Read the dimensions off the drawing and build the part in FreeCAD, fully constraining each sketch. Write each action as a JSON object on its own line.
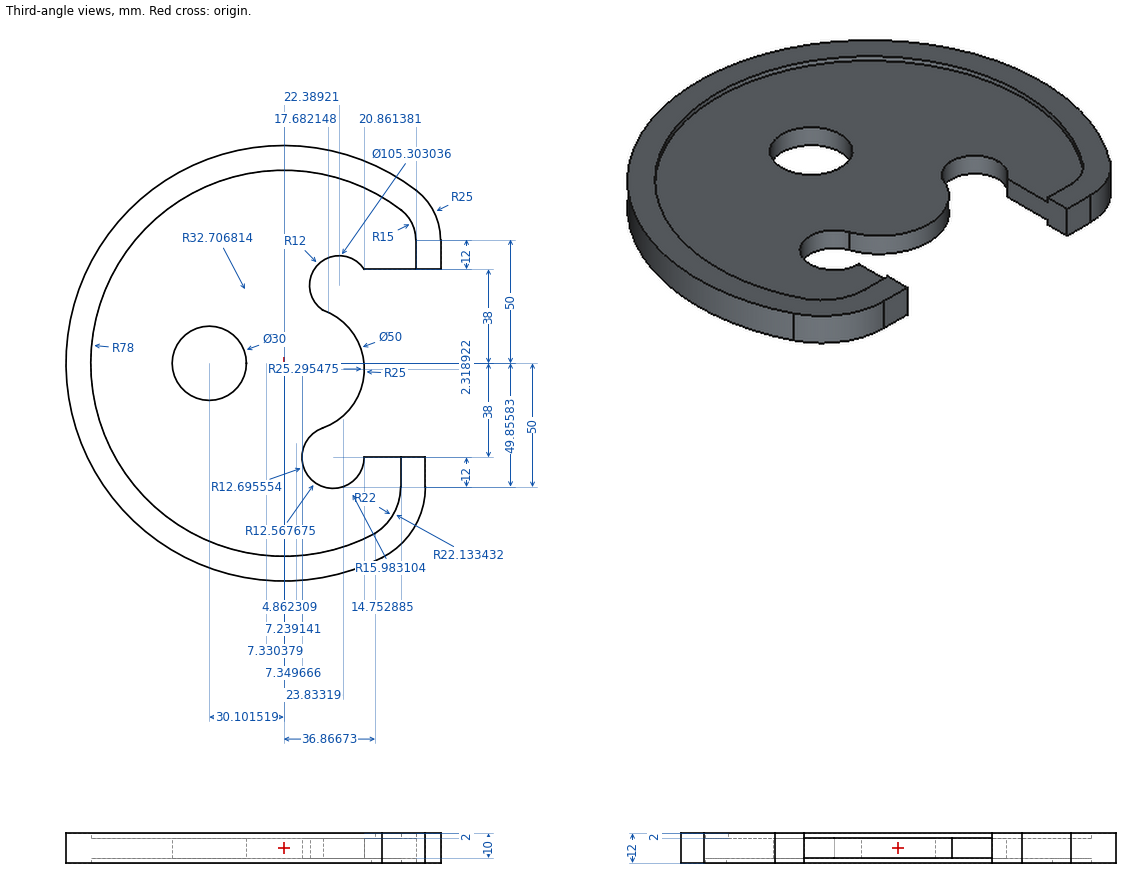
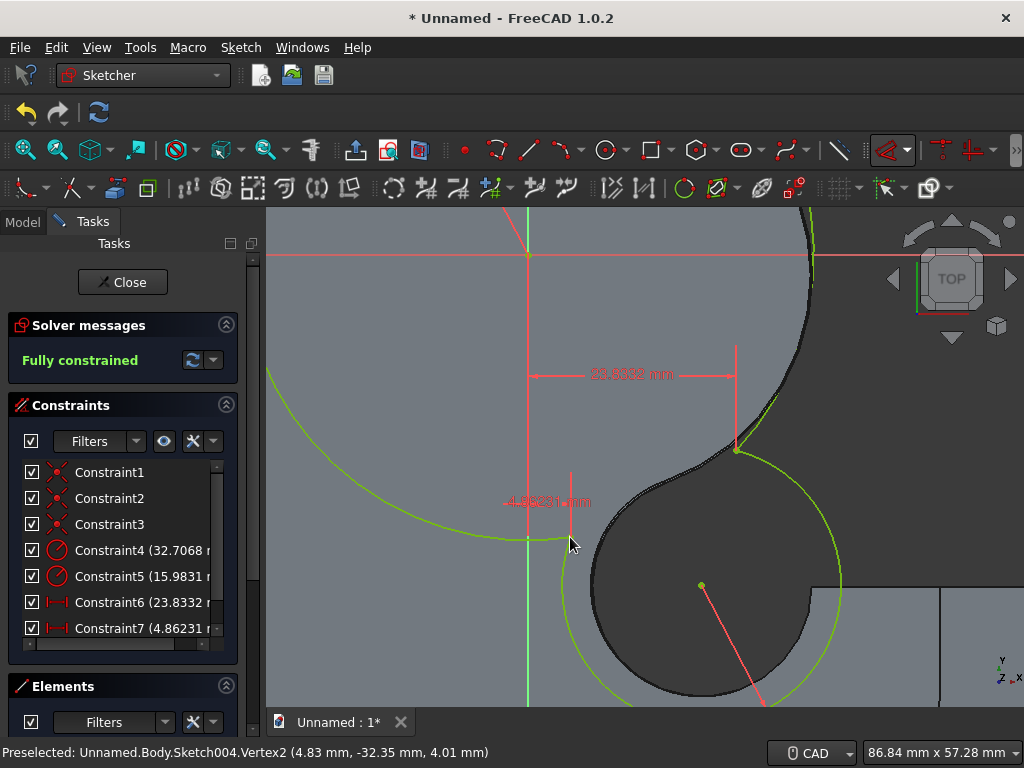
{"action": "left_click", "coordinate": [123, 282]}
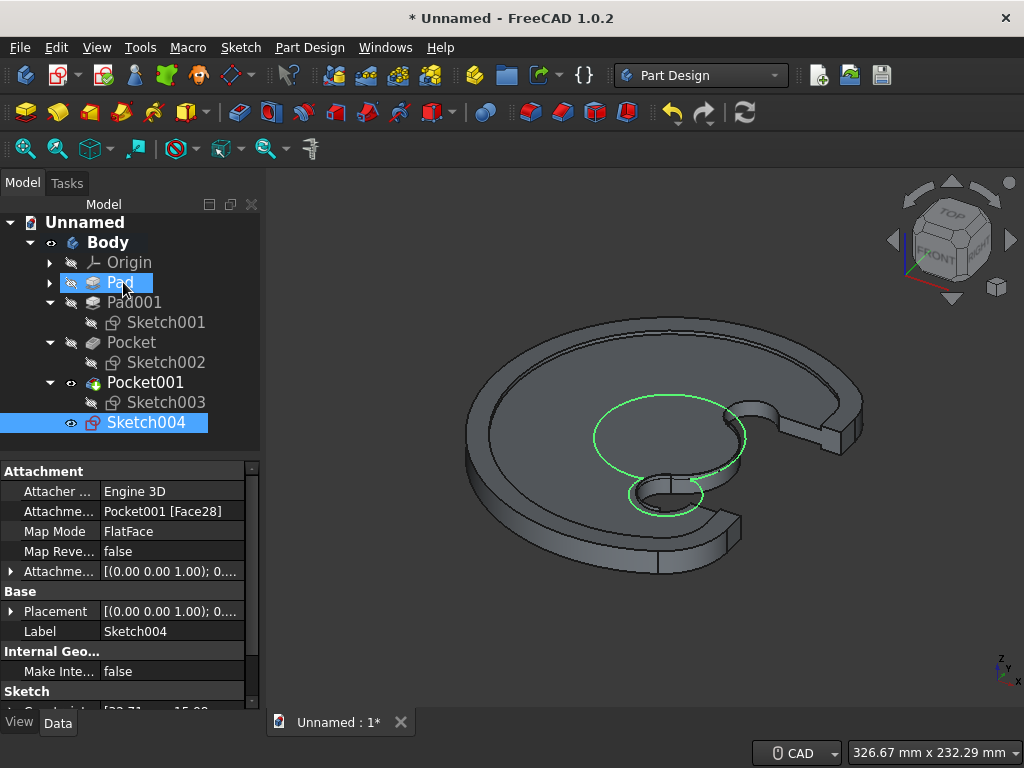
{"action": "left_click", "coordinate": [240, 112]}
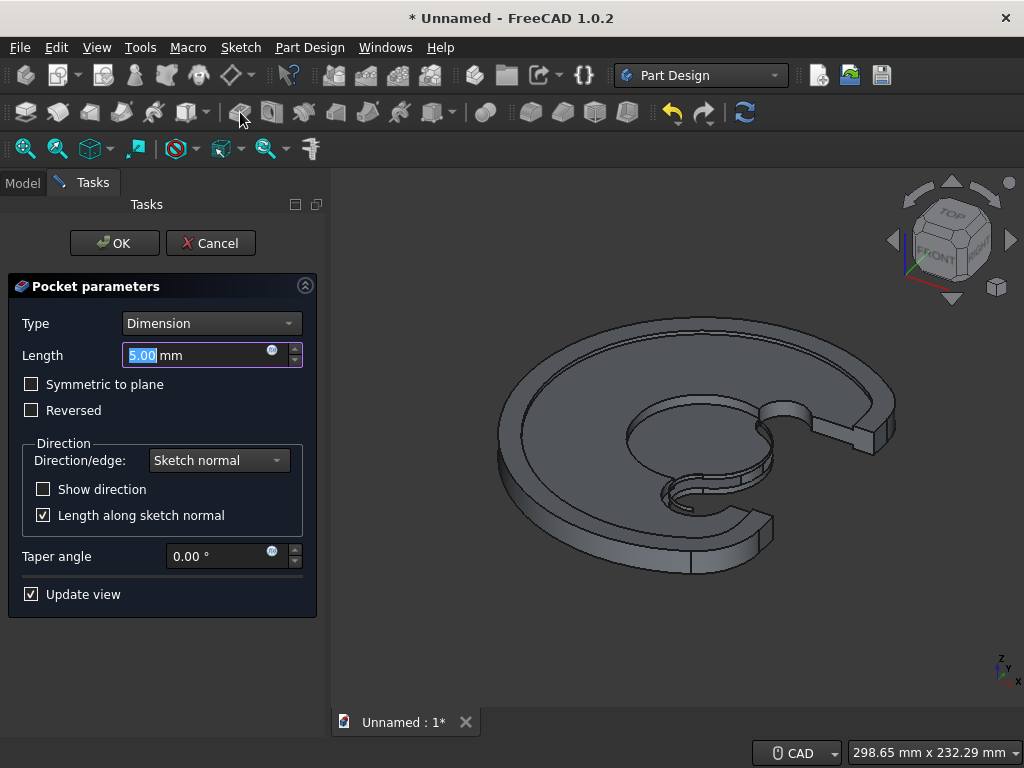
{"action": "type", "text": "2"}
{"action": "key", "text": "Tab"}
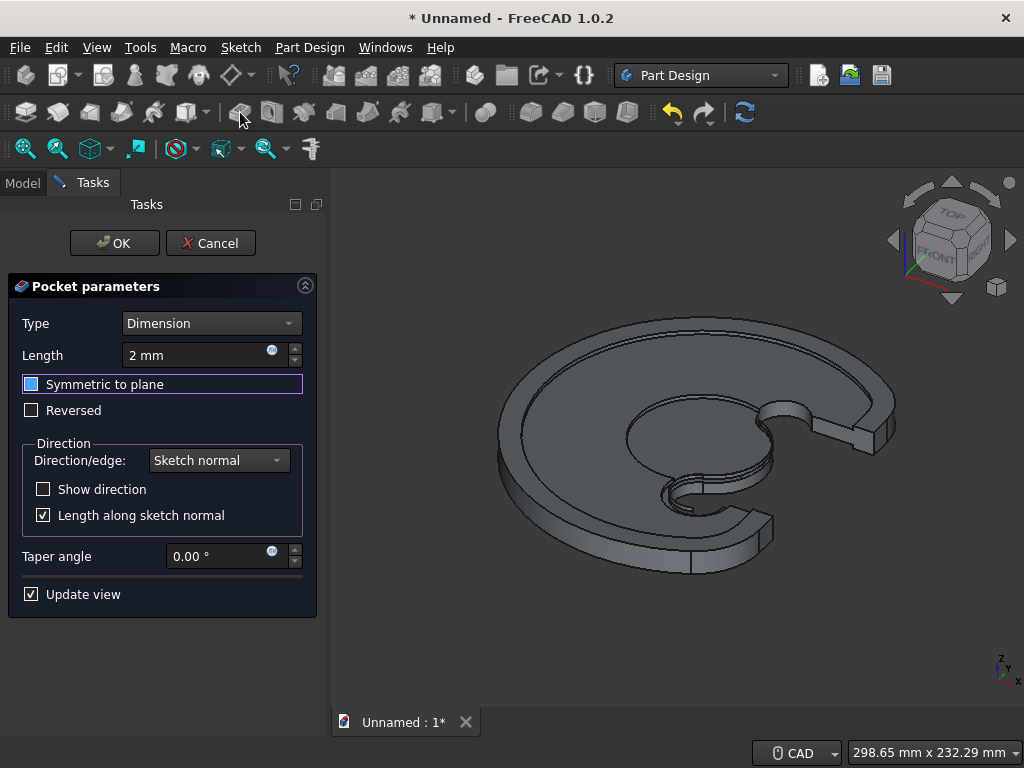
{"action": "left_click", "coordinate": [30, 410]}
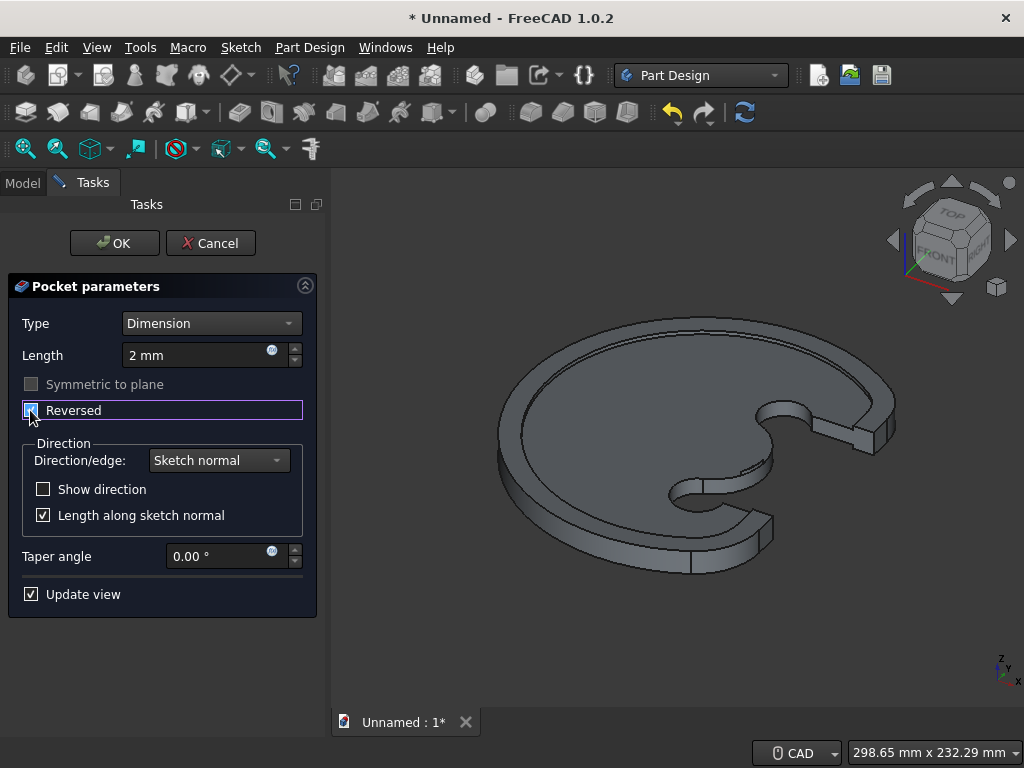
{"action": "left_click", "coordinate": [115, 243]}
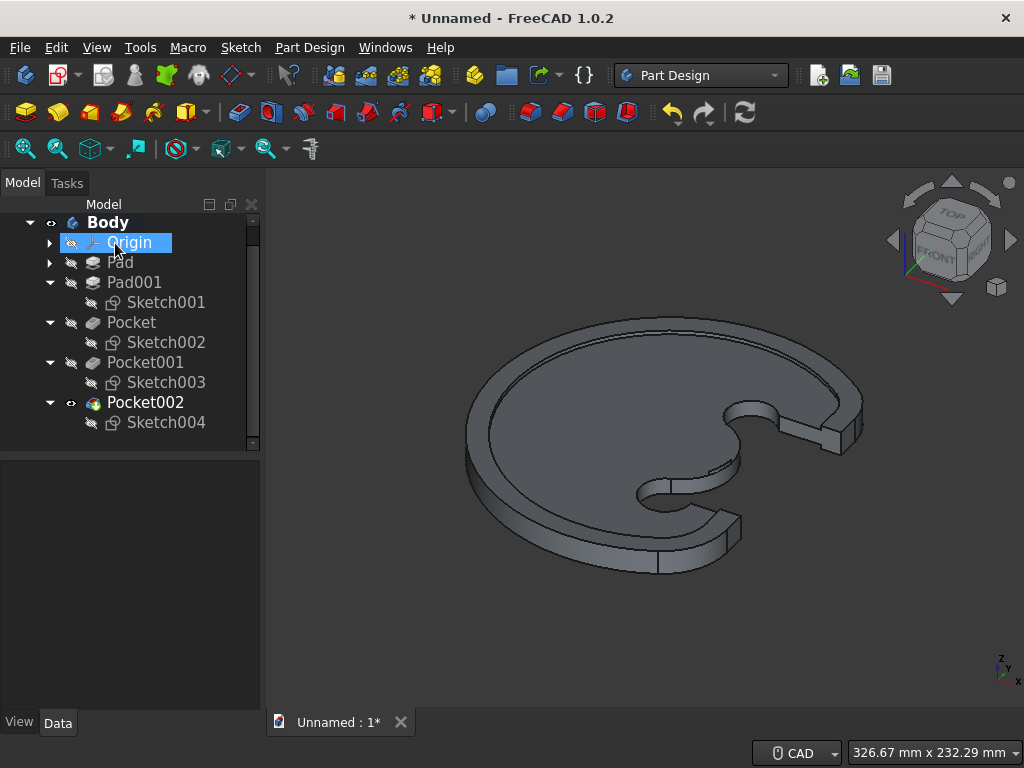
{"action": "left_click", "coordinate": [607, 416]}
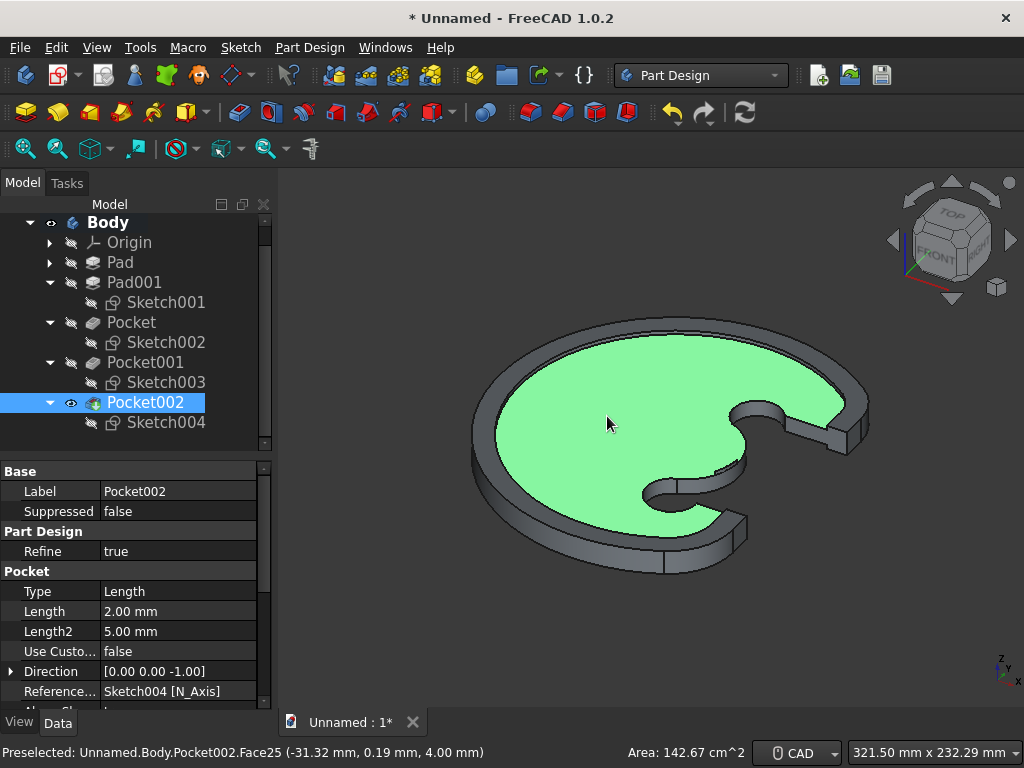
{"action": "left_click", "coordinate": [58, 76]}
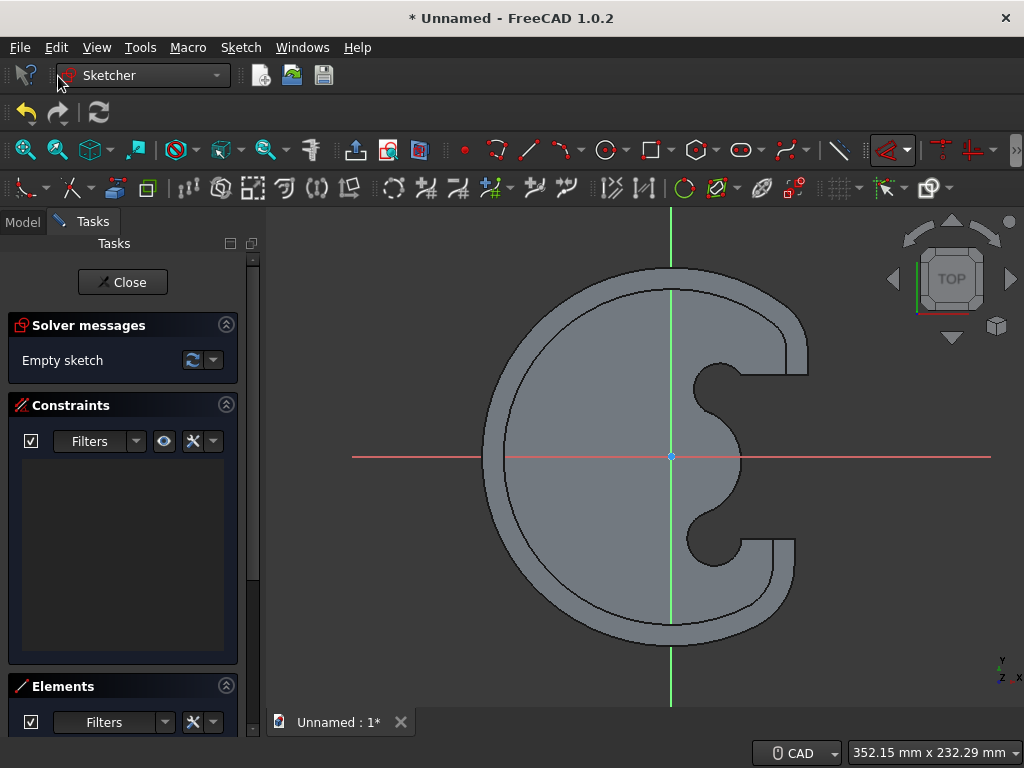
{"action": "scroll", "coordinate": [817, 457], "scroll_direction": "up", "scroll_amount": 2}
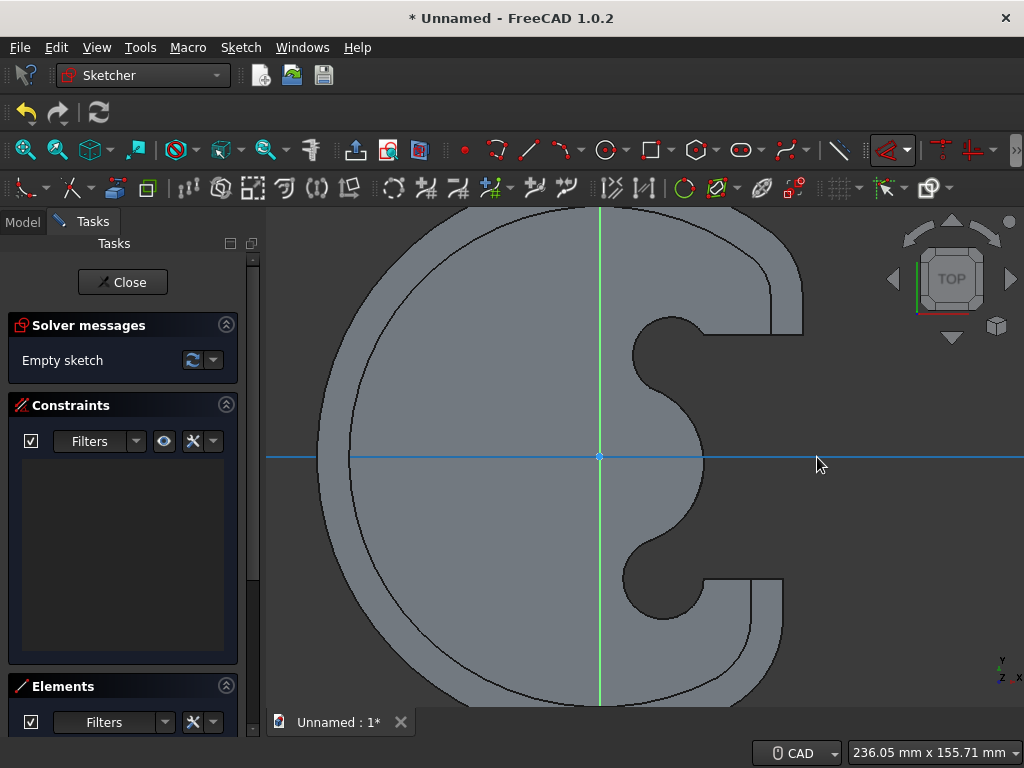
{"action": "left_click", "coordinate": [606, 150]}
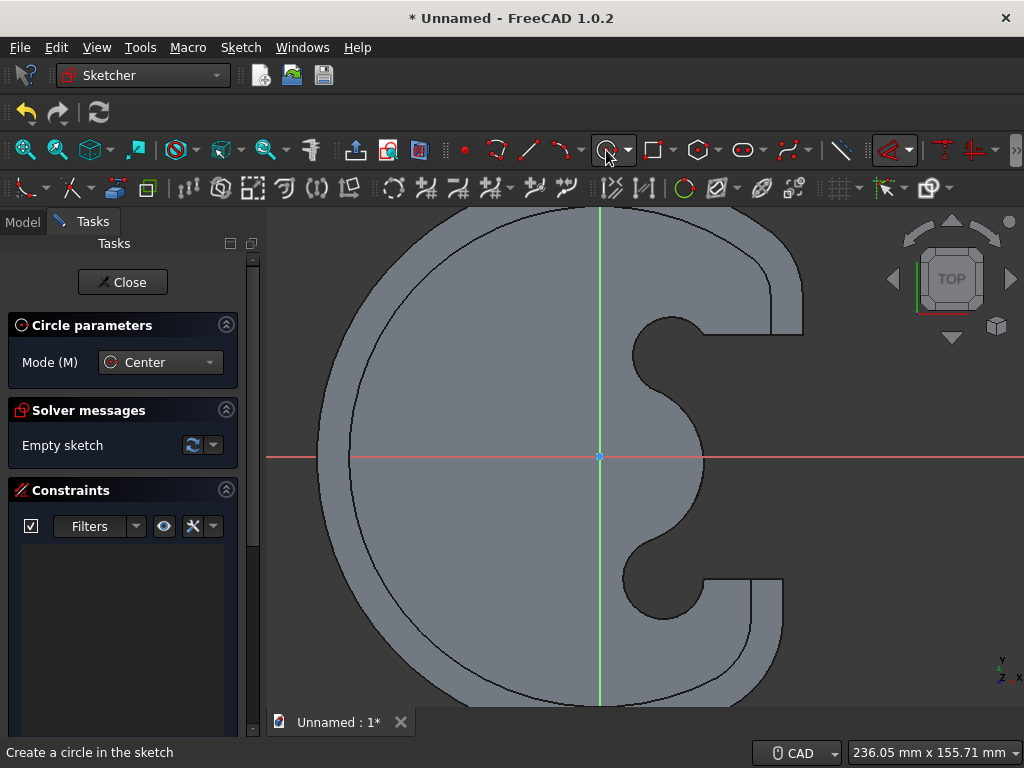
{"action": "left_click", "coordinate": [576, 457]}
{"action": "left_click", "coordinate": [696, 337]}
{"action": "key", "text": "Escape"}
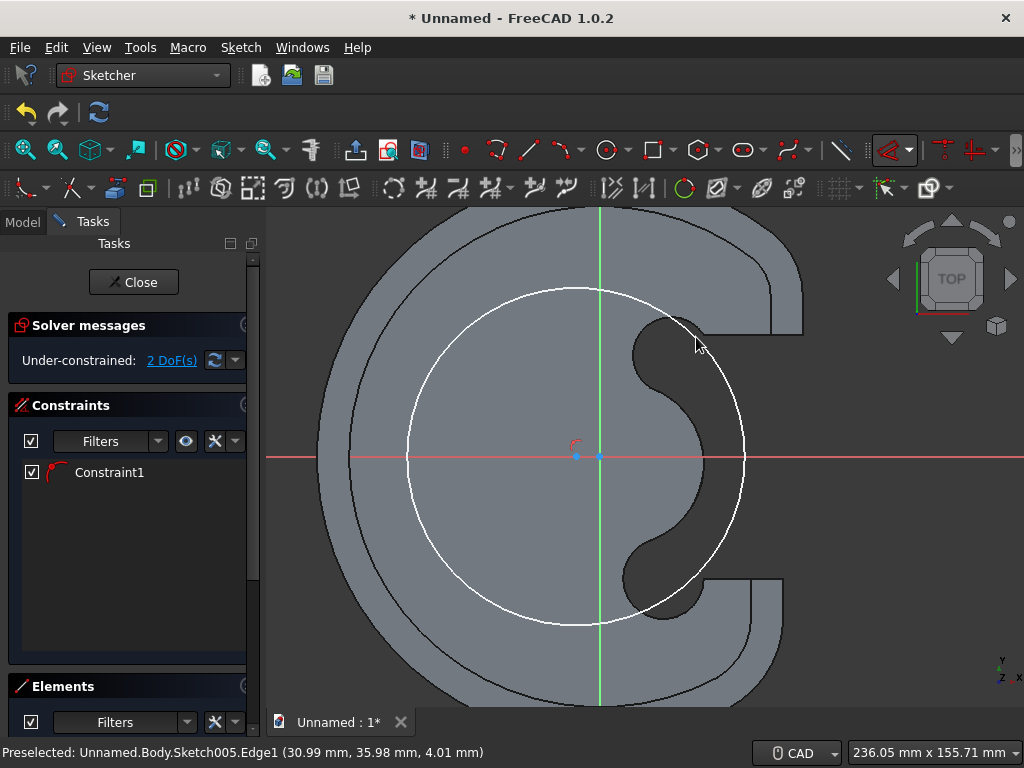
{"action": "left_click", "coordinate": [695, 337]}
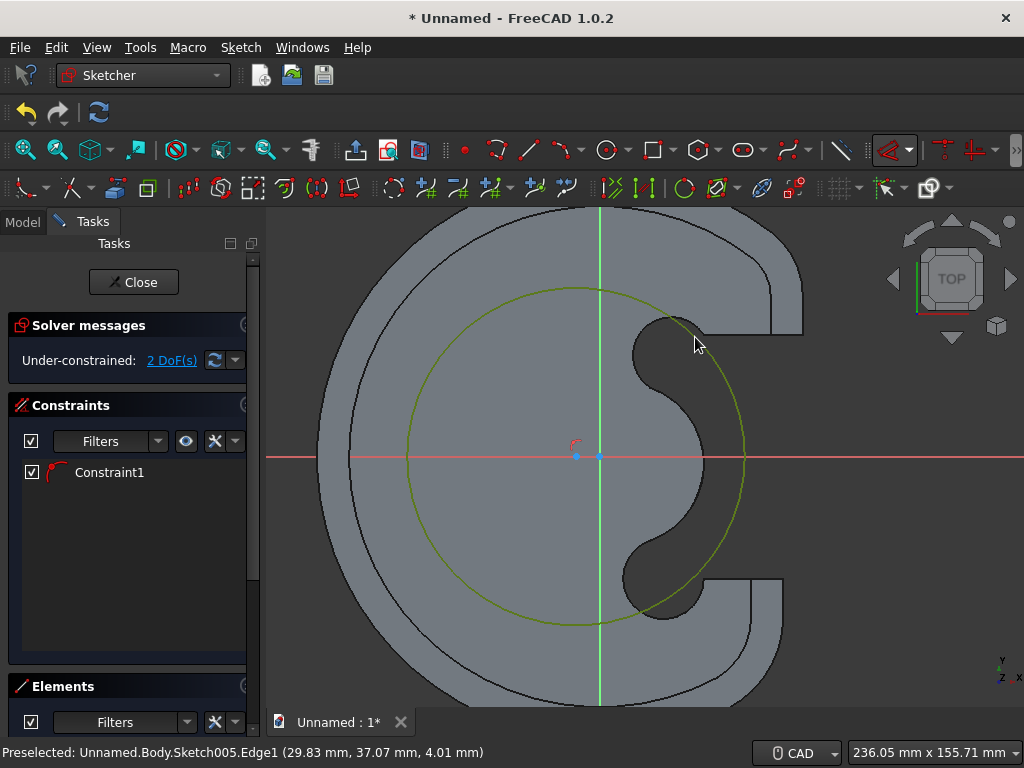
{"action": "key", "text": "k o"}